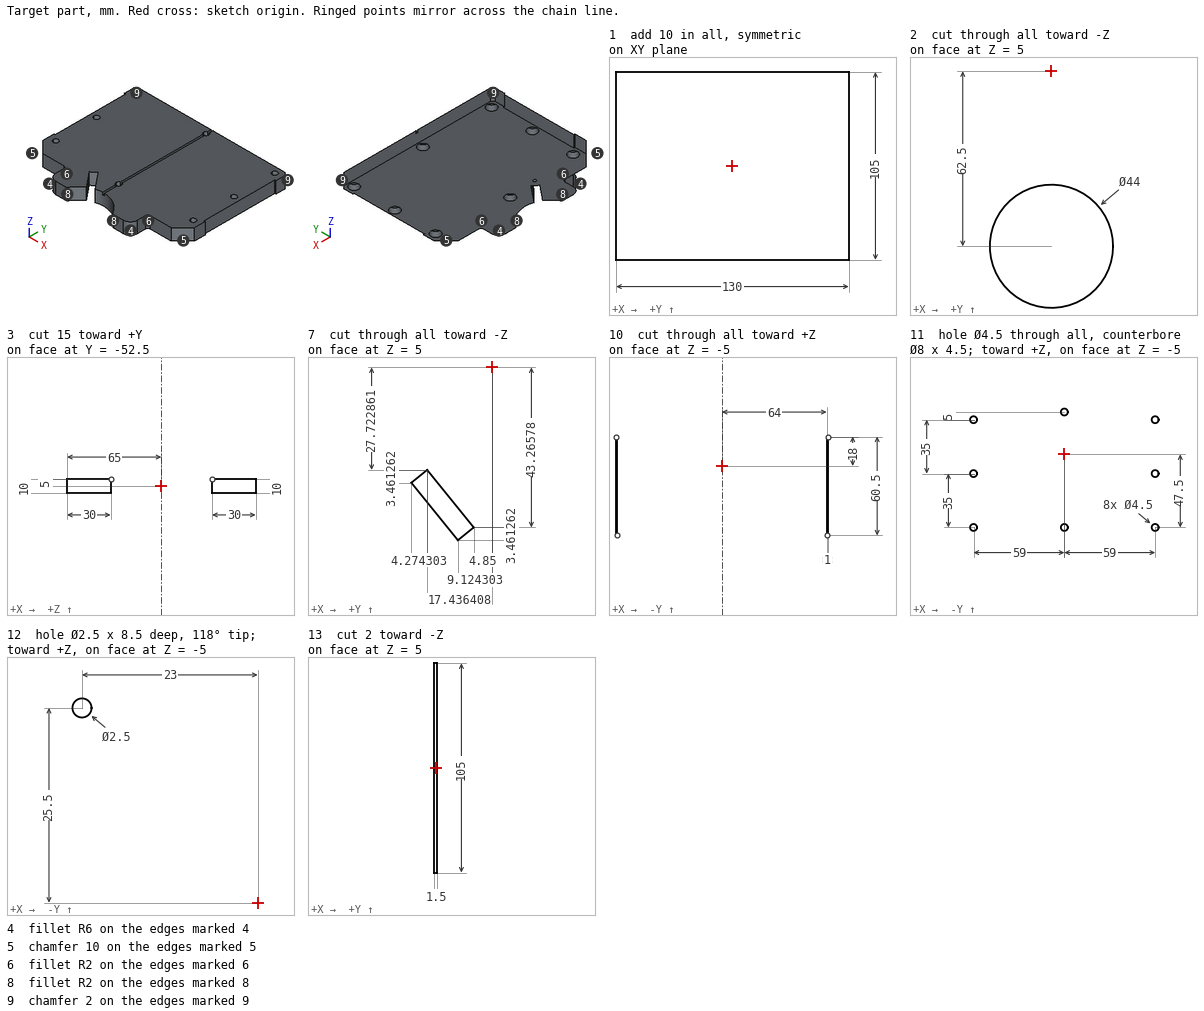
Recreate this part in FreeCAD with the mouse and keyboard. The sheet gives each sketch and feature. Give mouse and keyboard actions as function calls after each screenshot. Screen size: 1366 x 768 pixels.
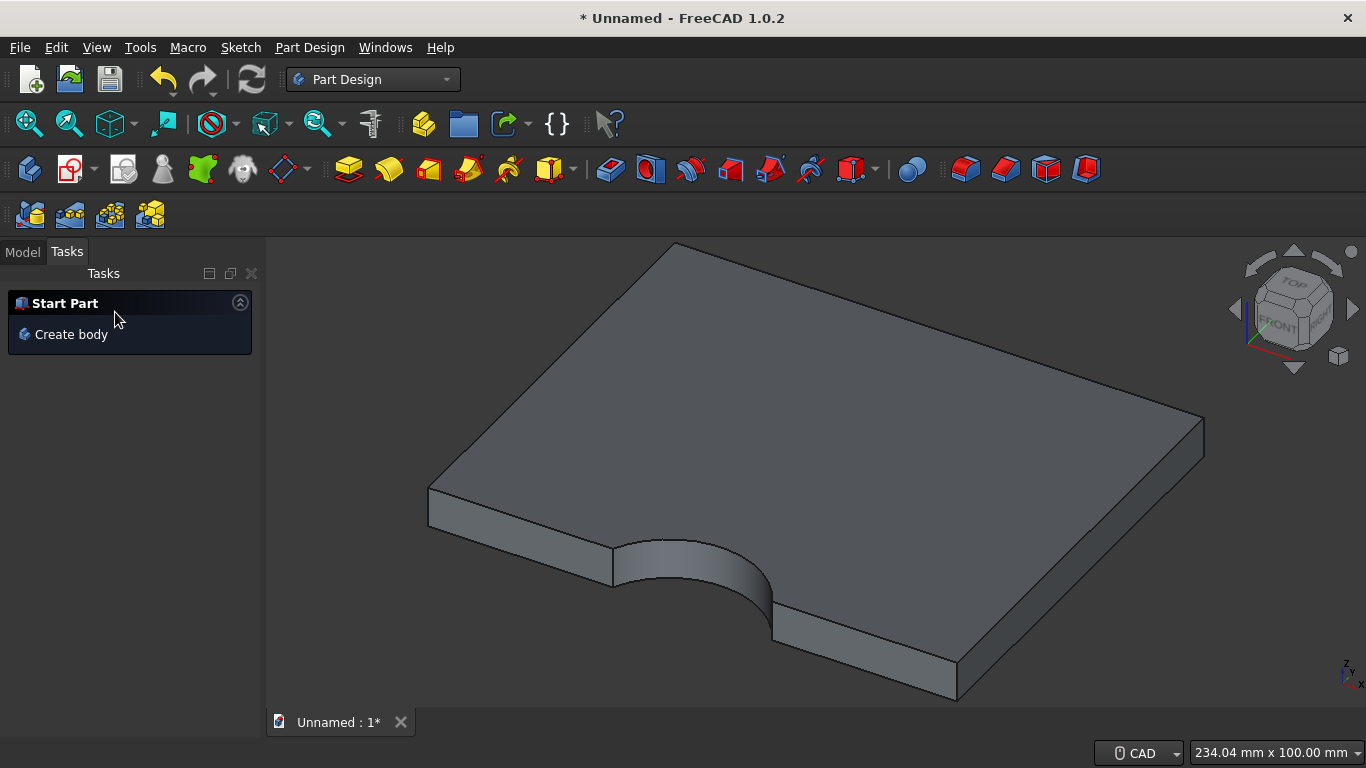
click(918, 668)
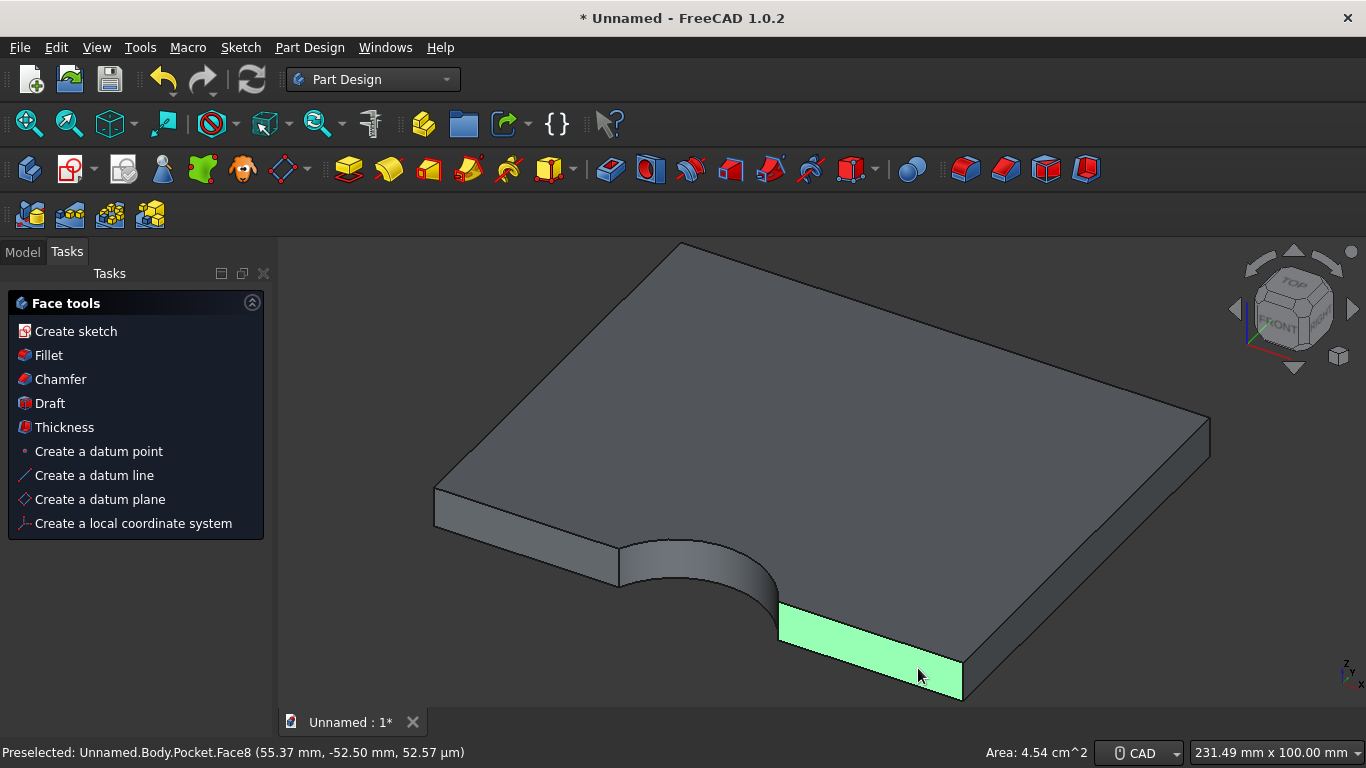
click(70, 170)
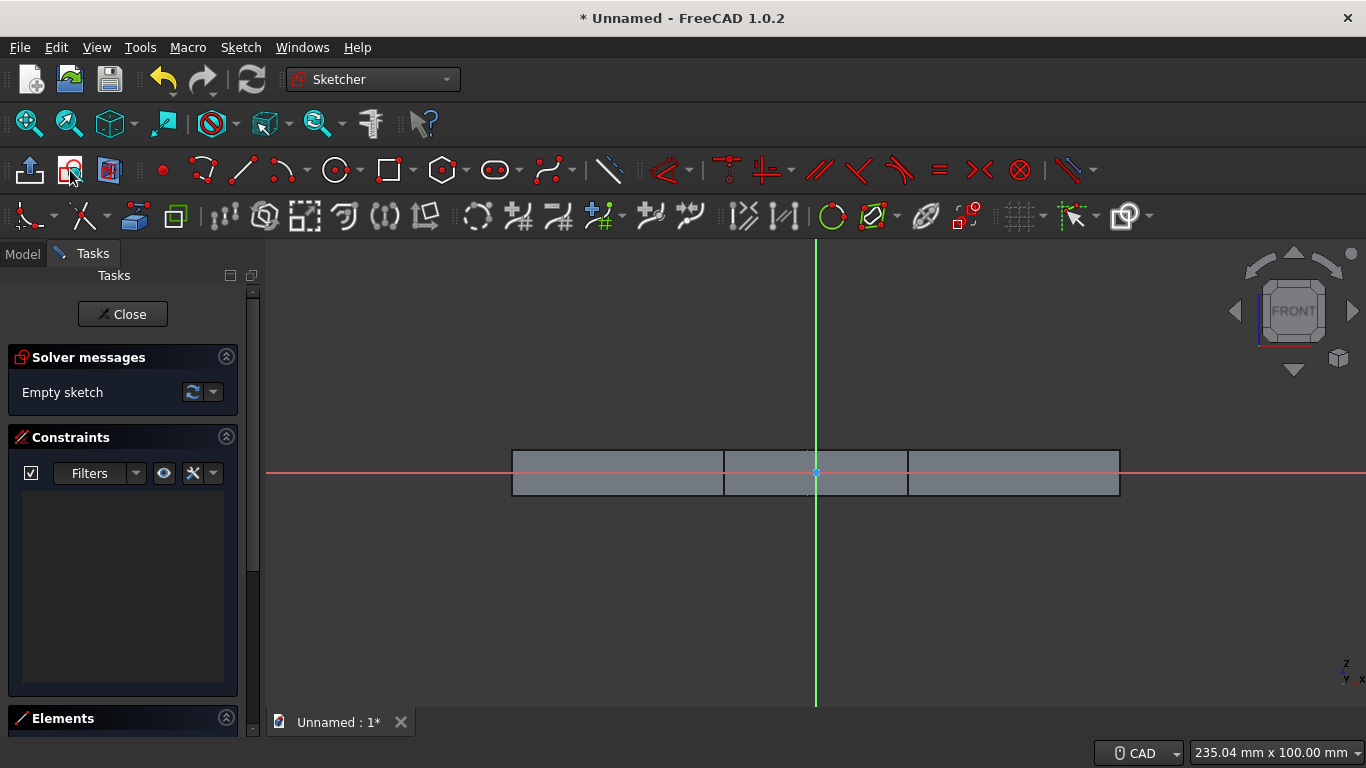
click(390, 170)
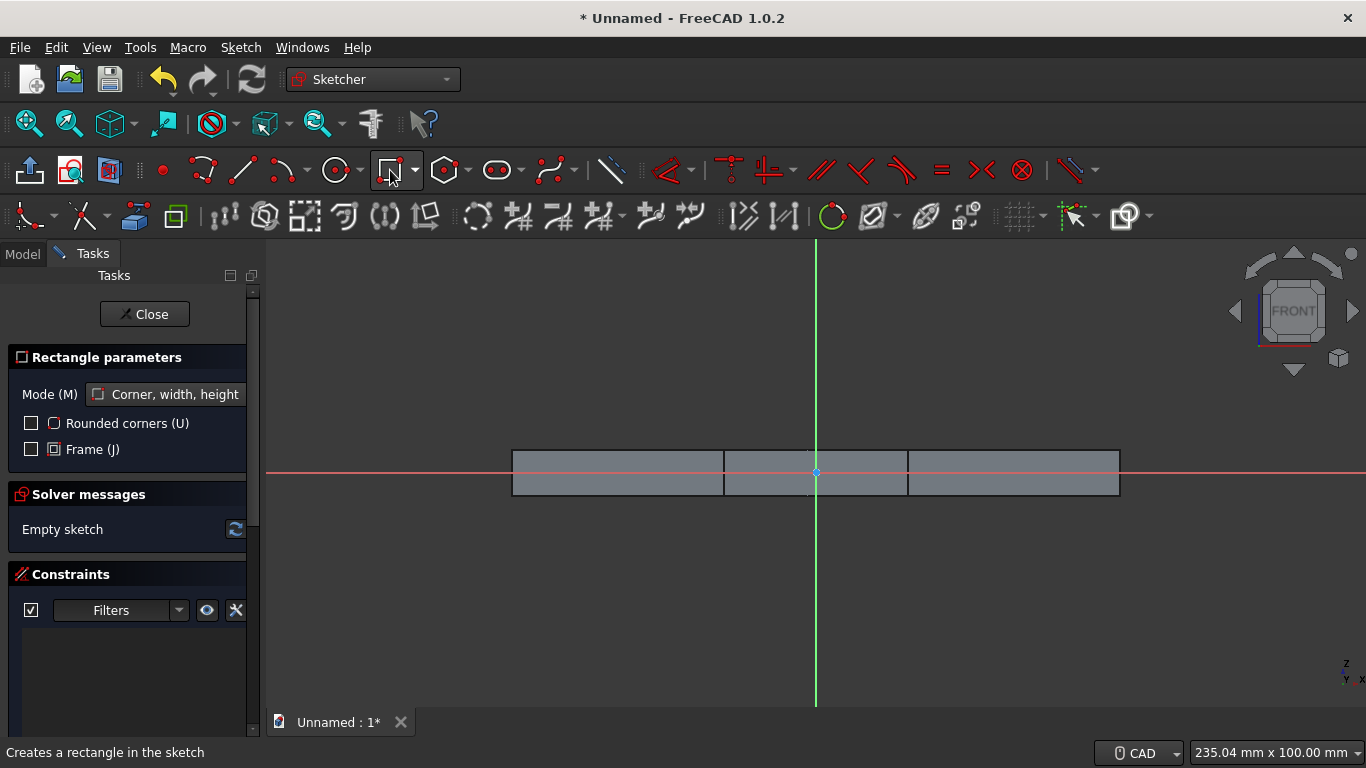
click(512, 450)
move(652, 496)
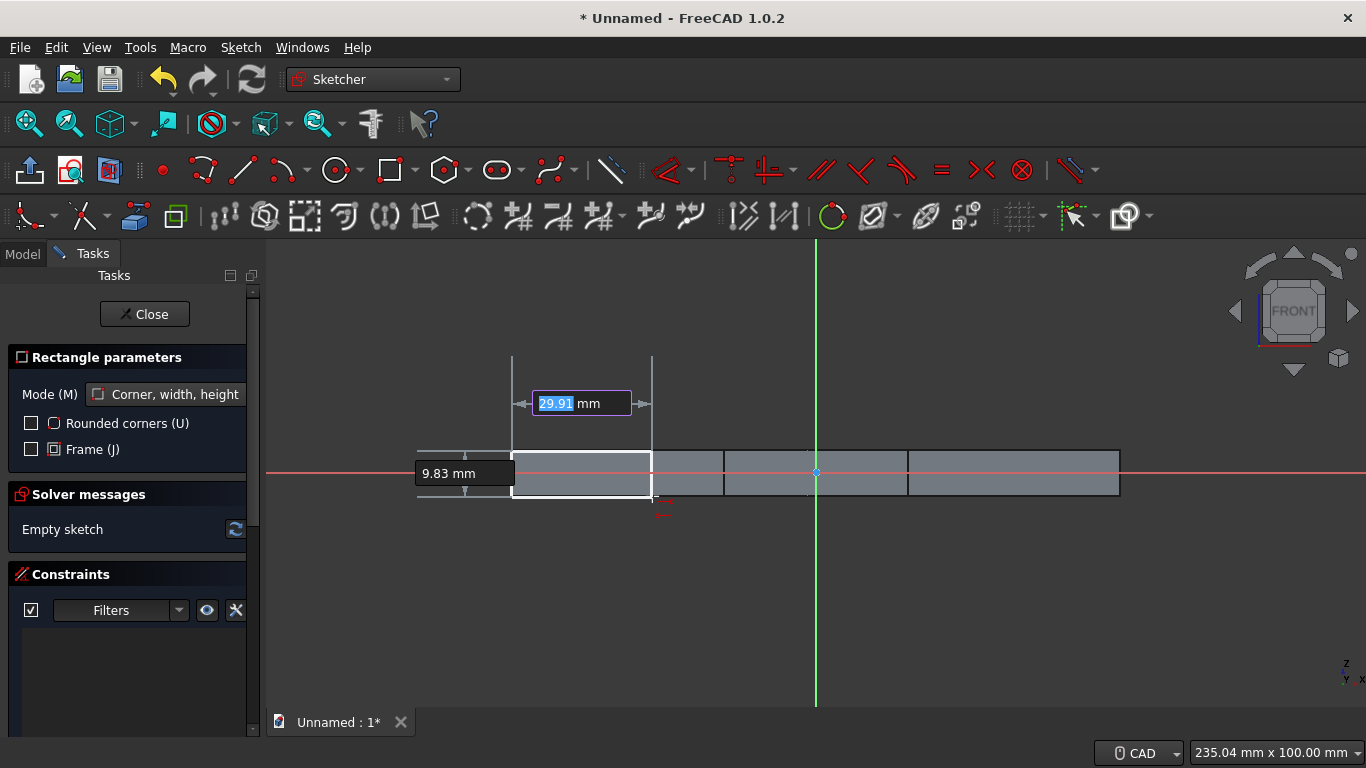
text(30)
key(Tab)
text(10)
key(Return)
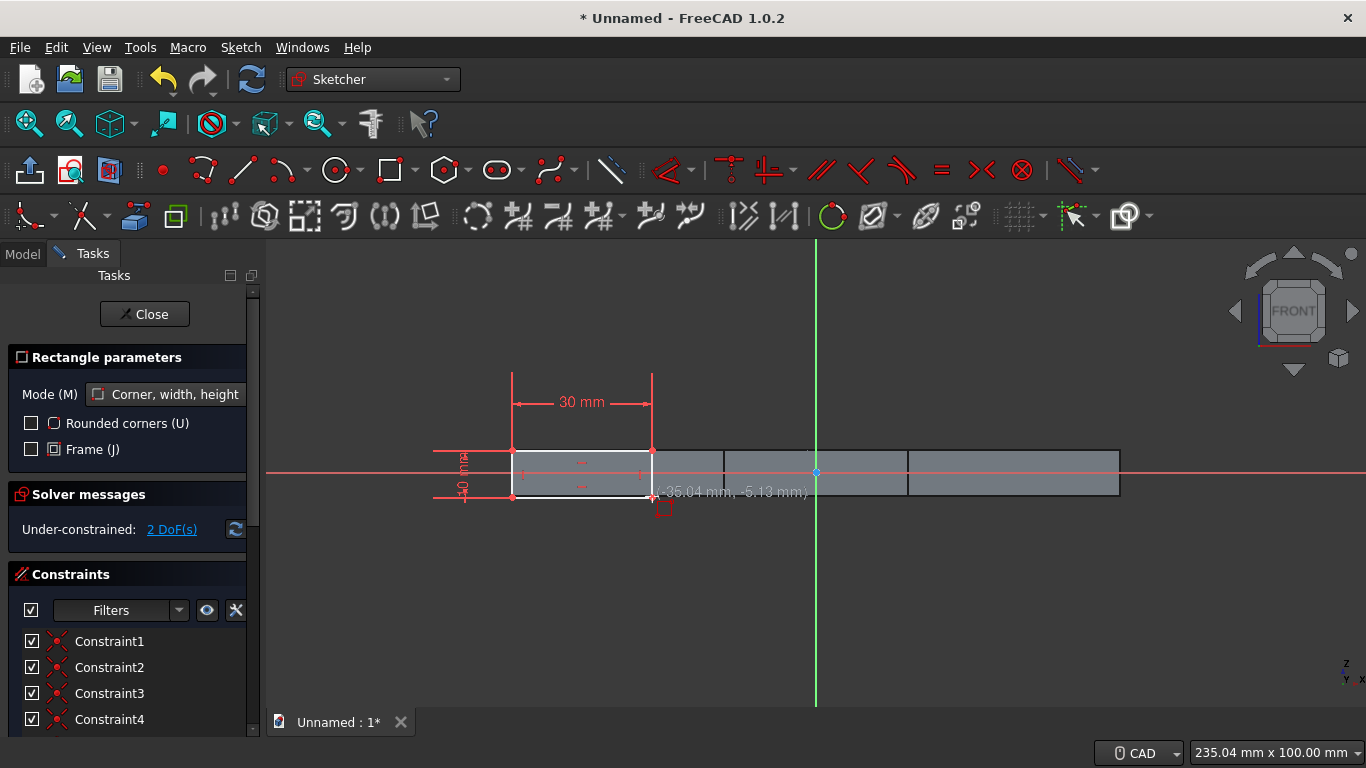
click(980, 450)
move(1120, 496)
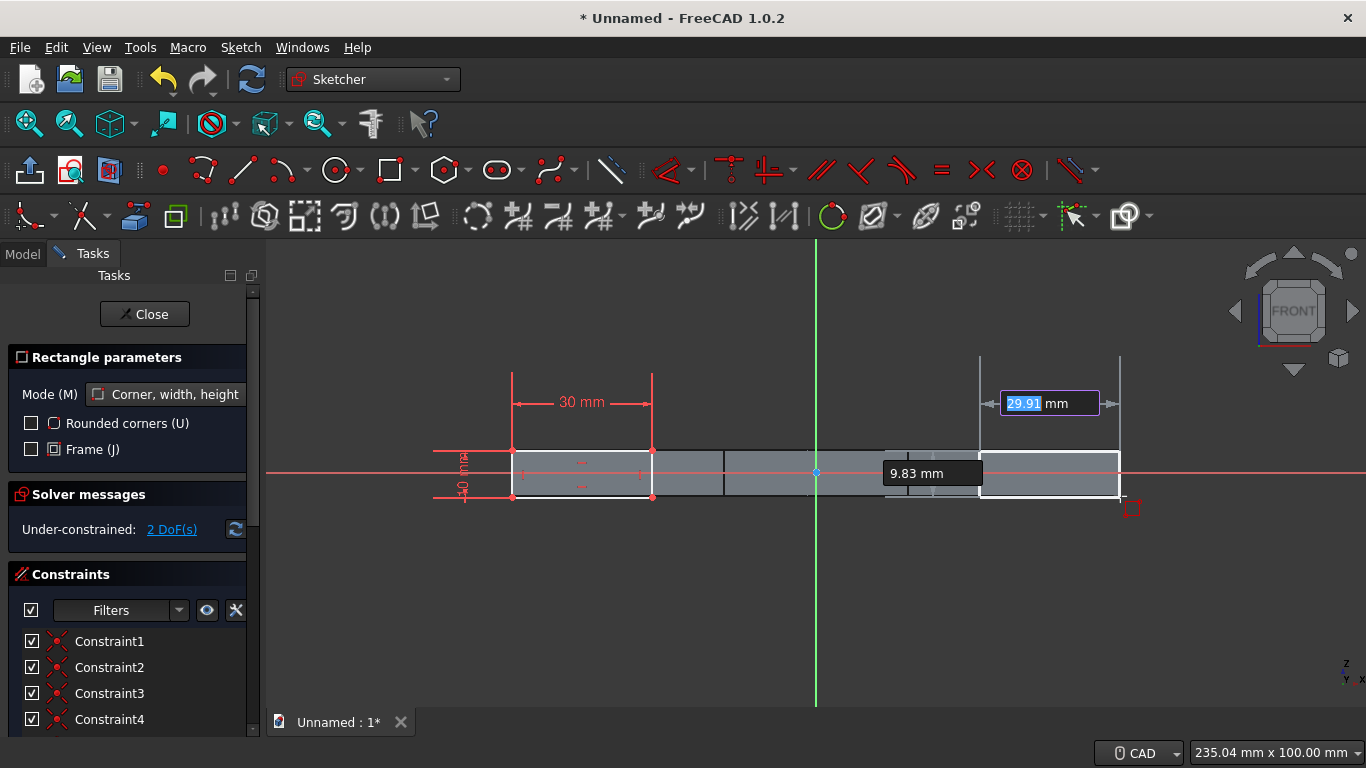
text(30)
key(Tab)
text(10)
key(Return)
key(Escape)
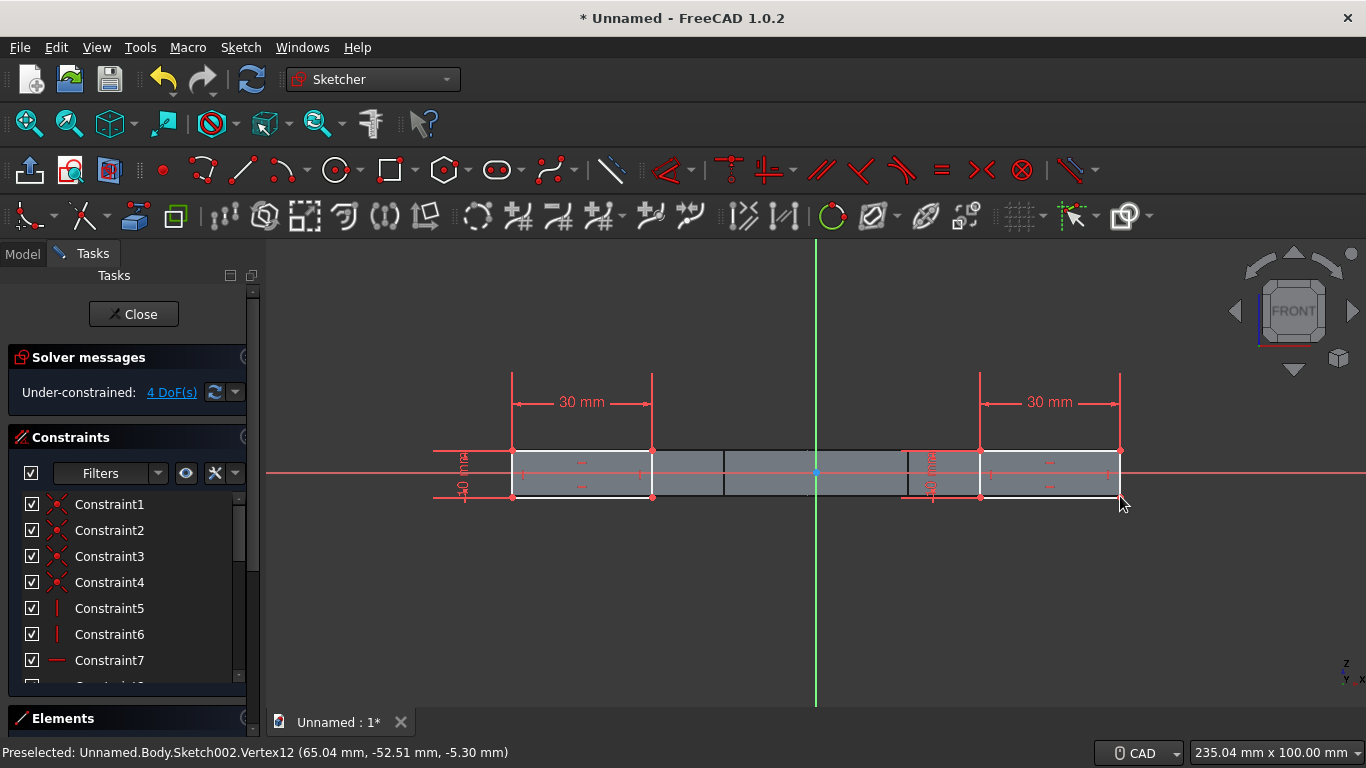
click(652, 451)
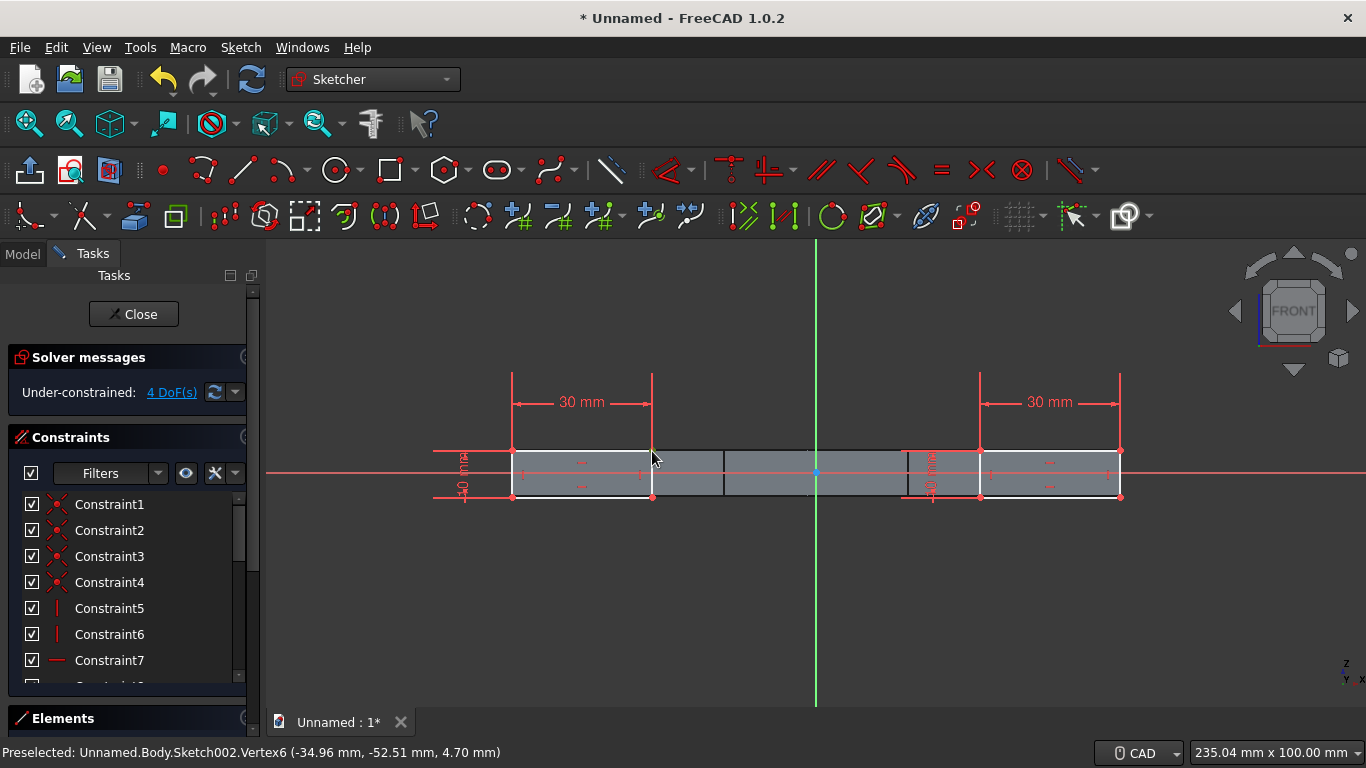
click(980, 451)